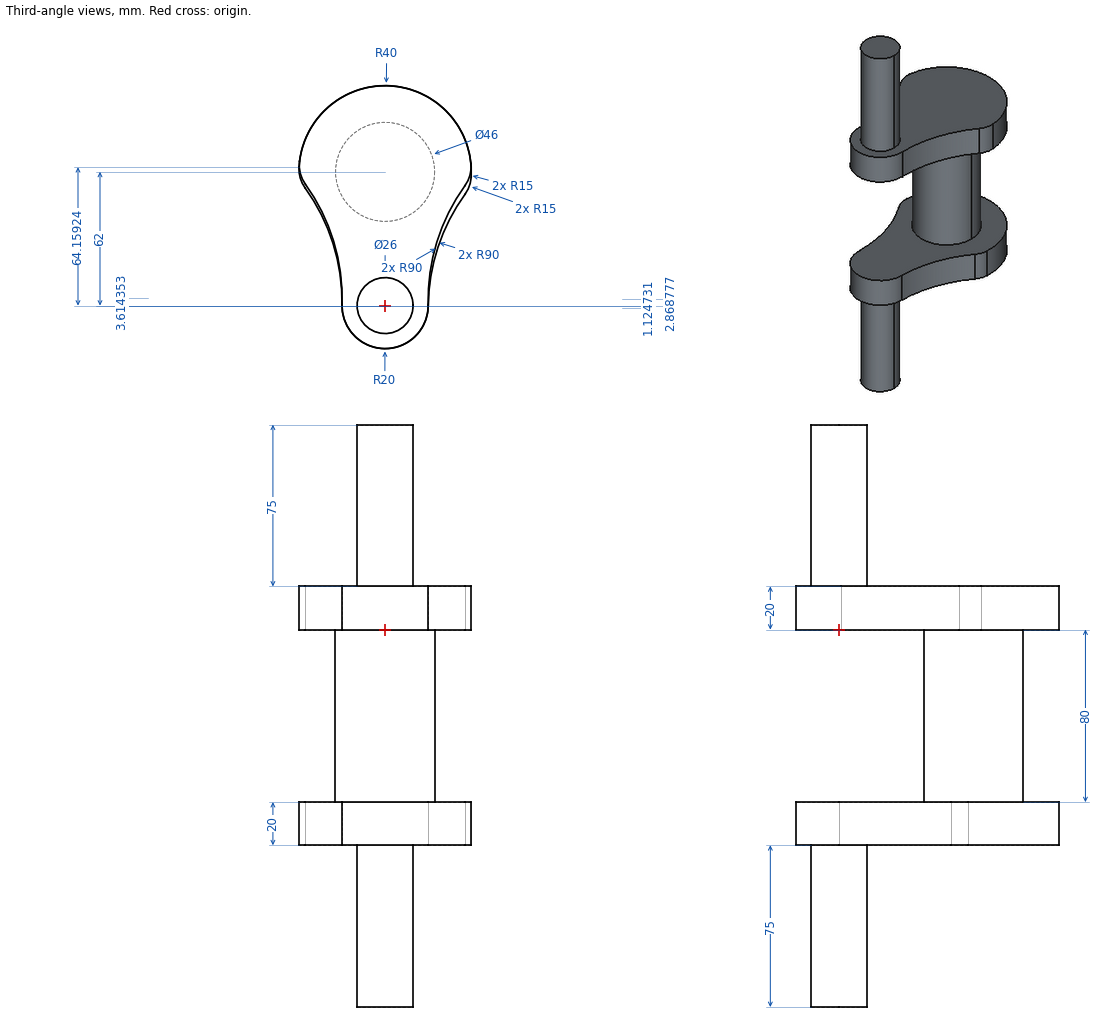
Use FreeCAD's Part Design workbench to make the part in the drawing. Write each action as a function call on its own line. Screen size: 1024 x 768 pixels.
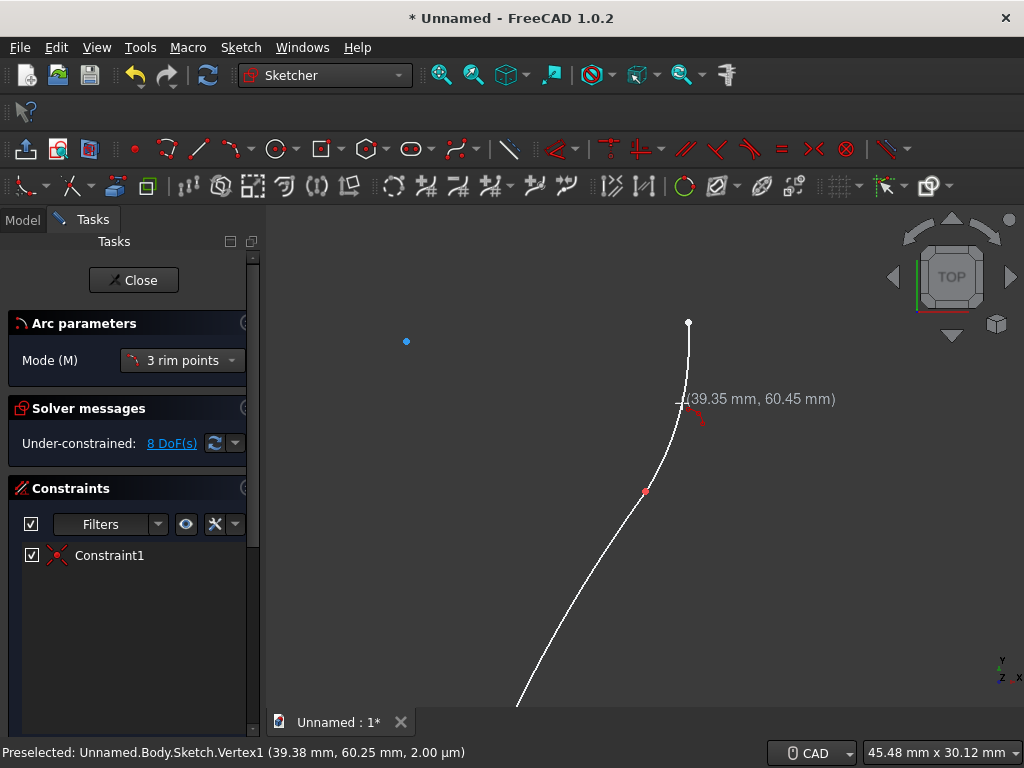
scroll(685, 402, down, 9)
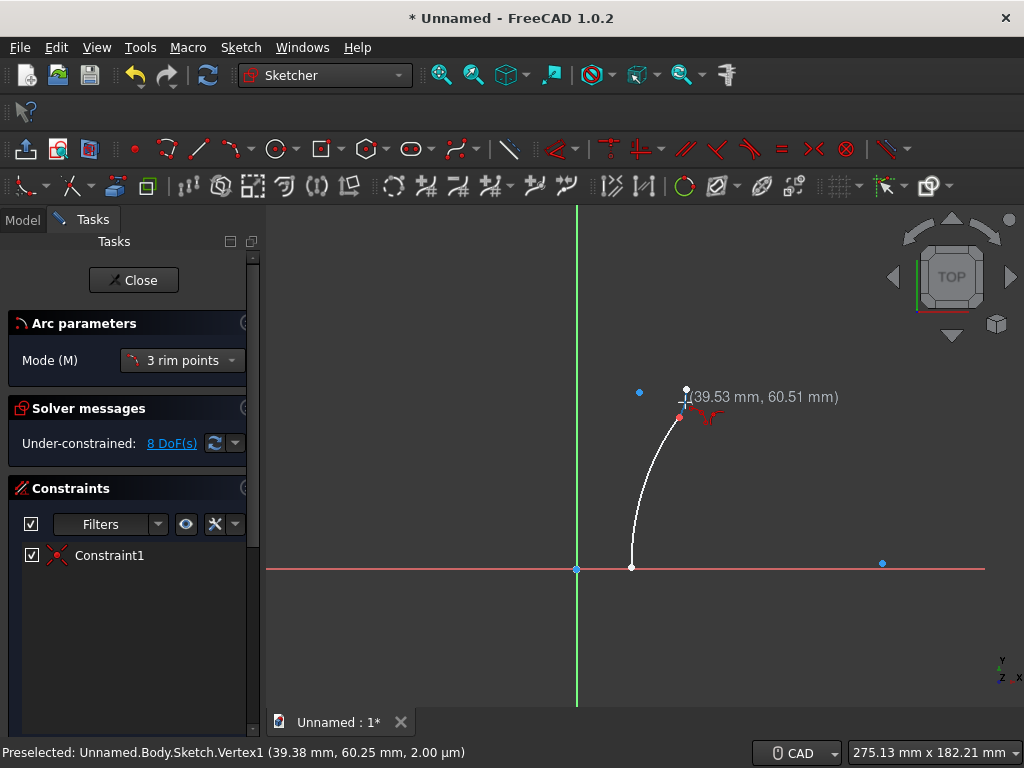
click(686, 389)
click(467, 385)
click(610, 293)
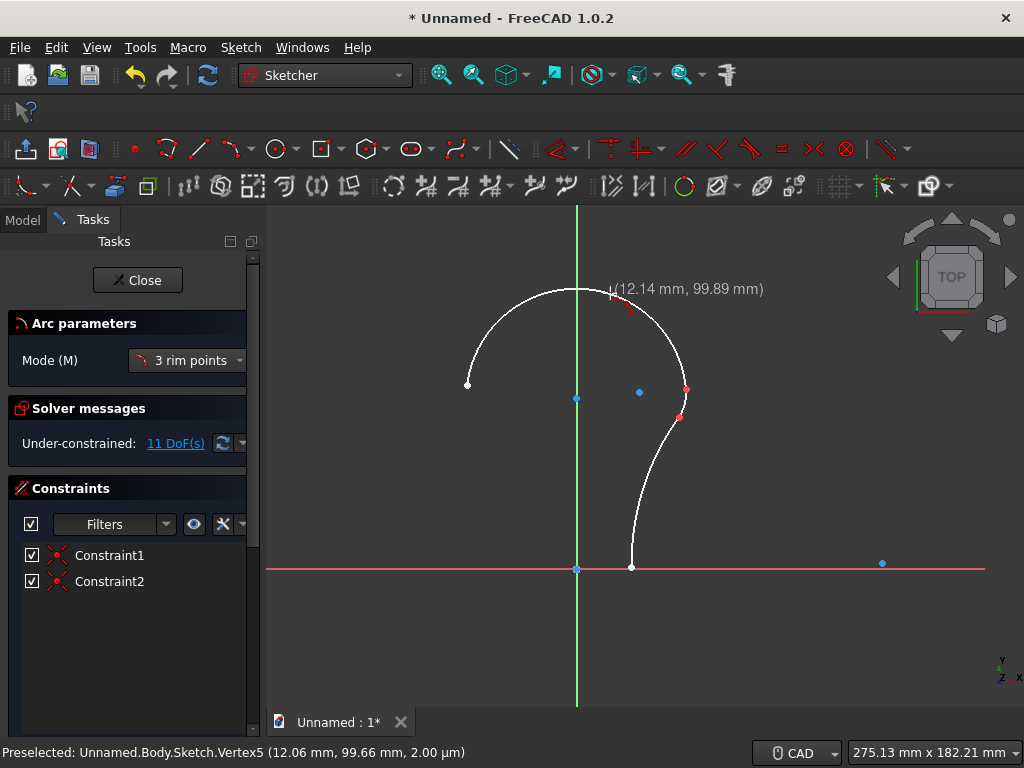
click(467, 386)
click(475, 414)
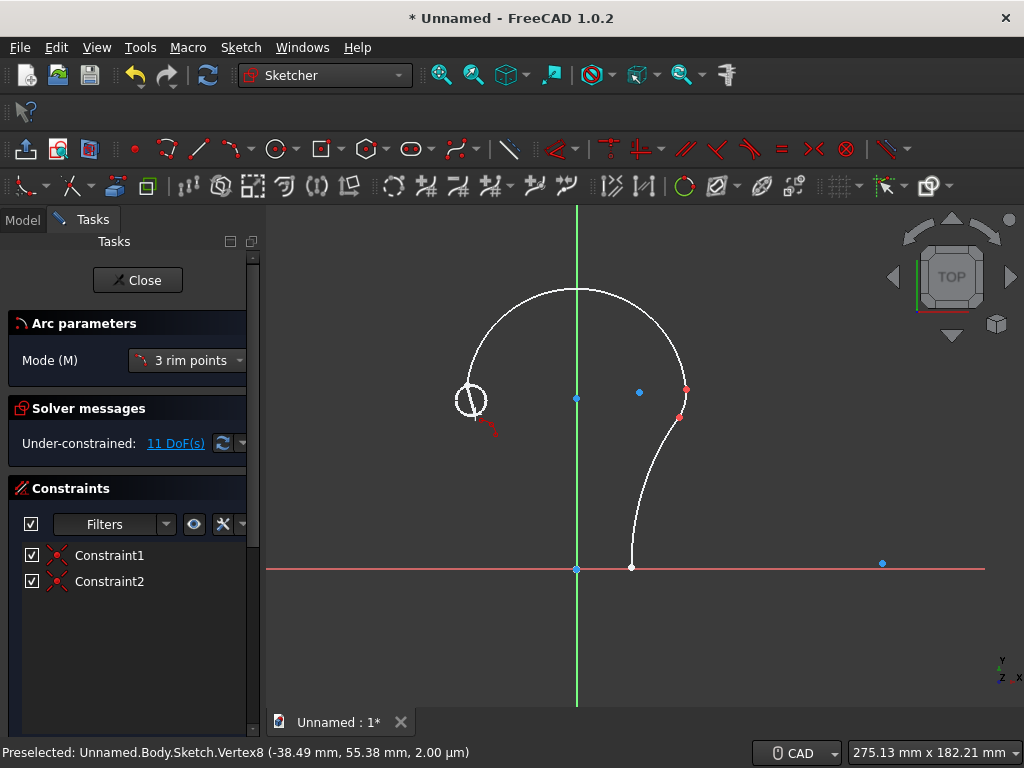
scroll(468, 400, up, 9)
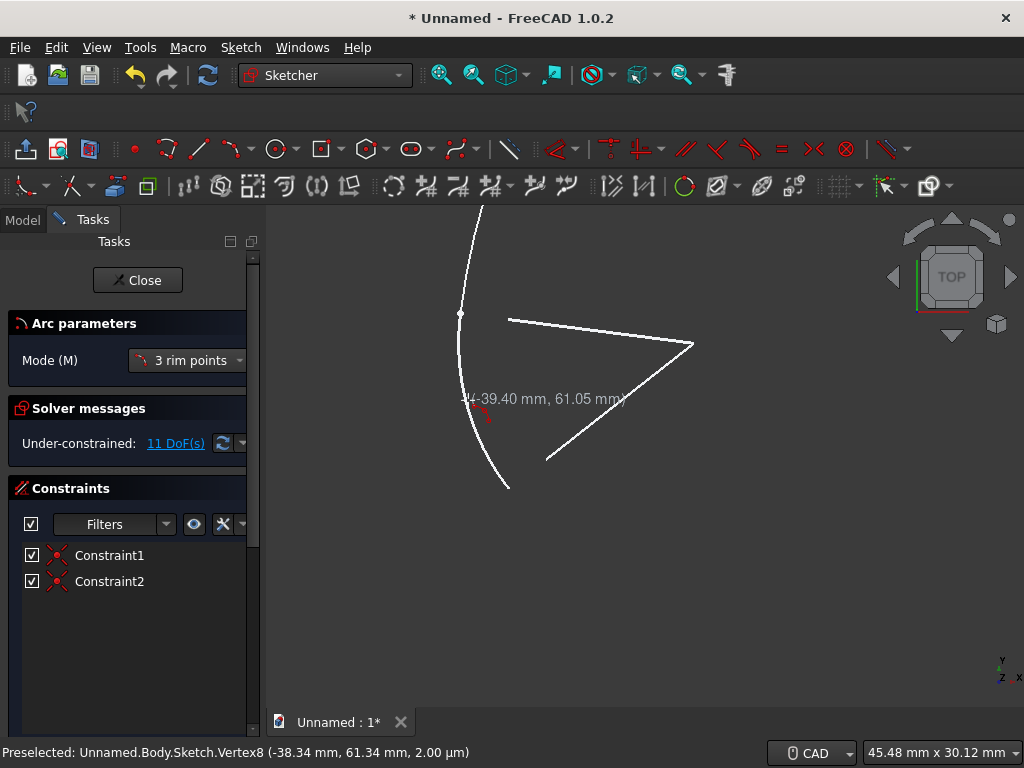
click(468, 399)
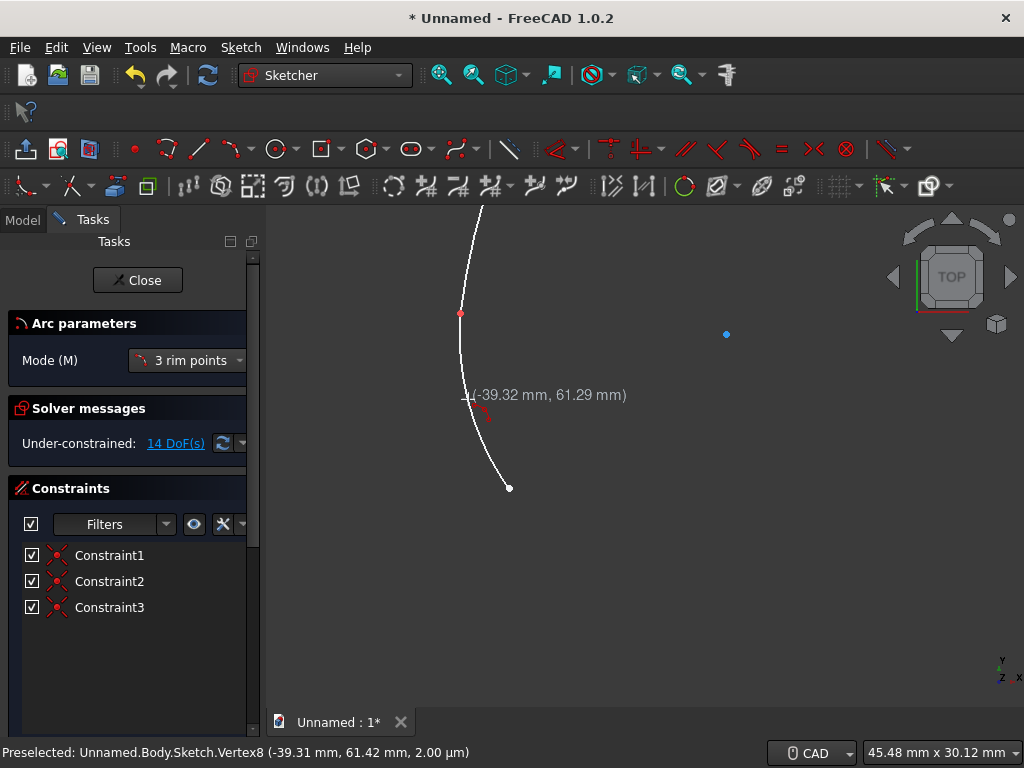
scroll(468, 400, down, 9)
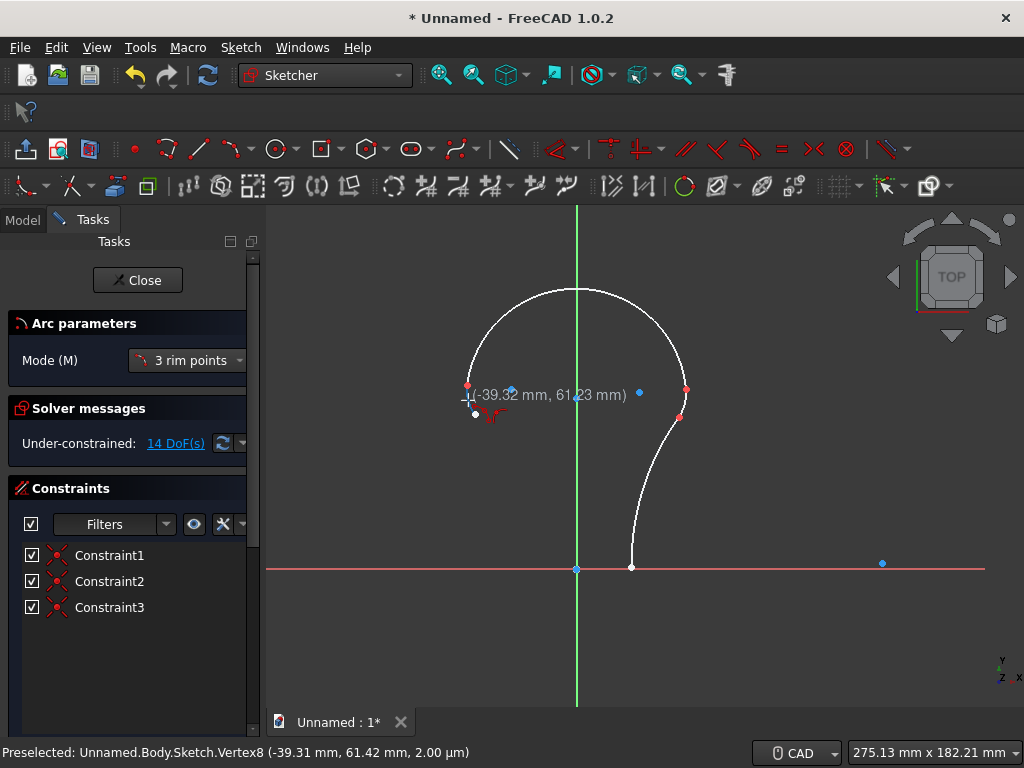
click(475, 415)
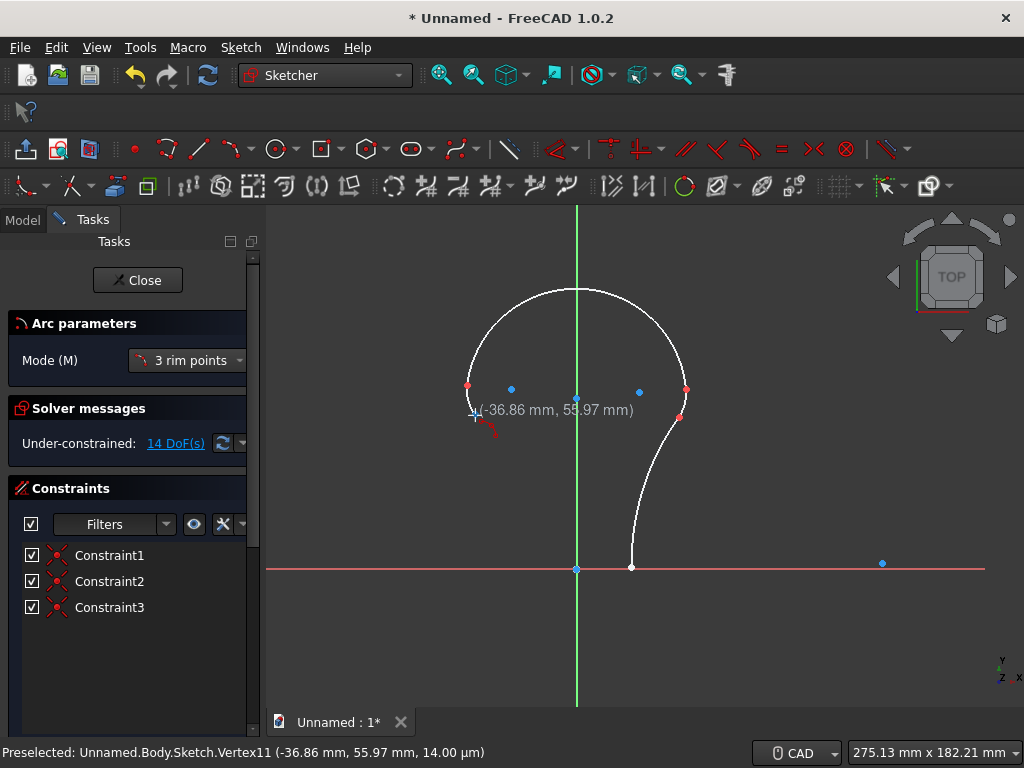
scroll(521, 567, up, 11)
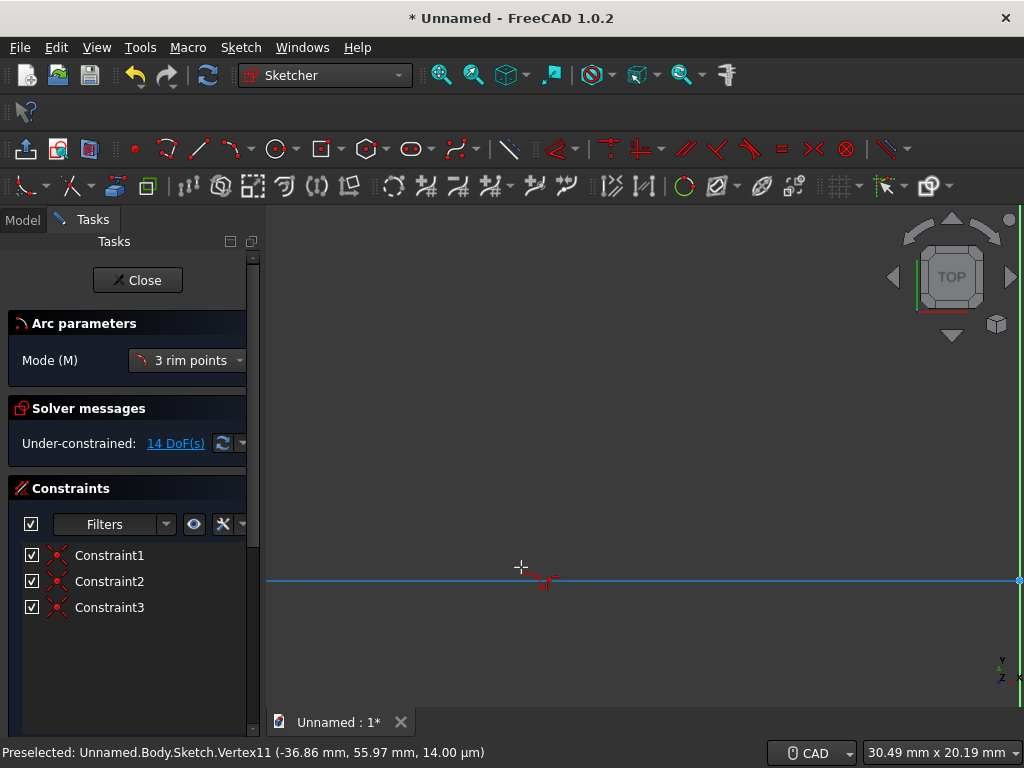
click(523, 565)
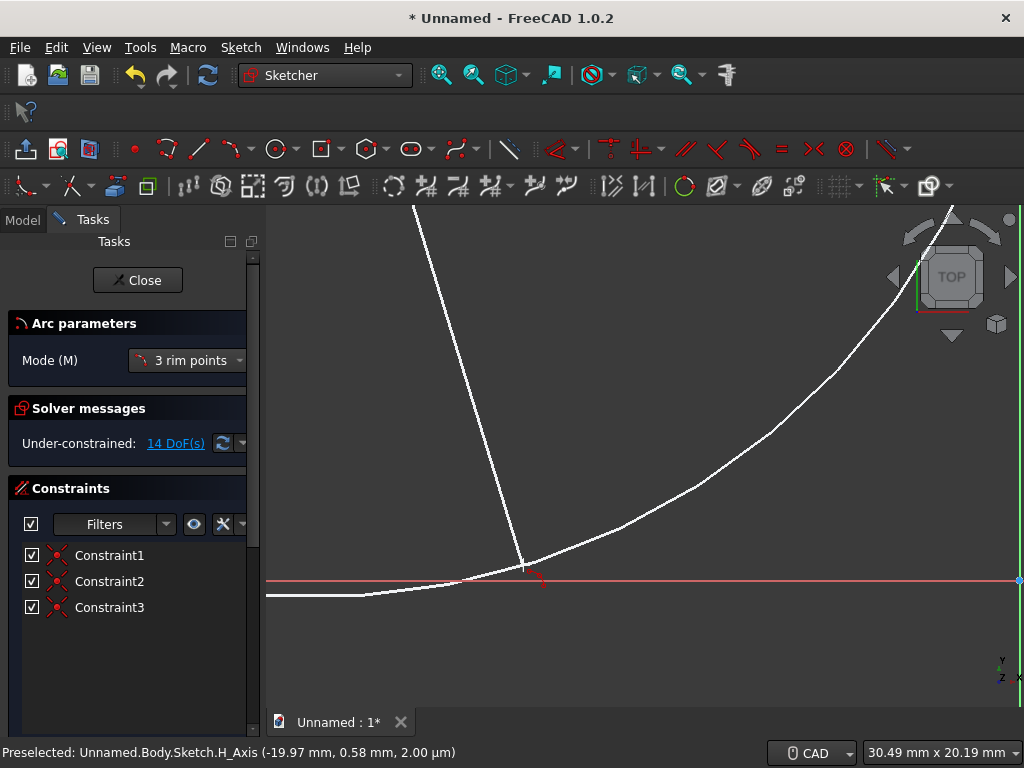
scroll(521, 567, down, 11)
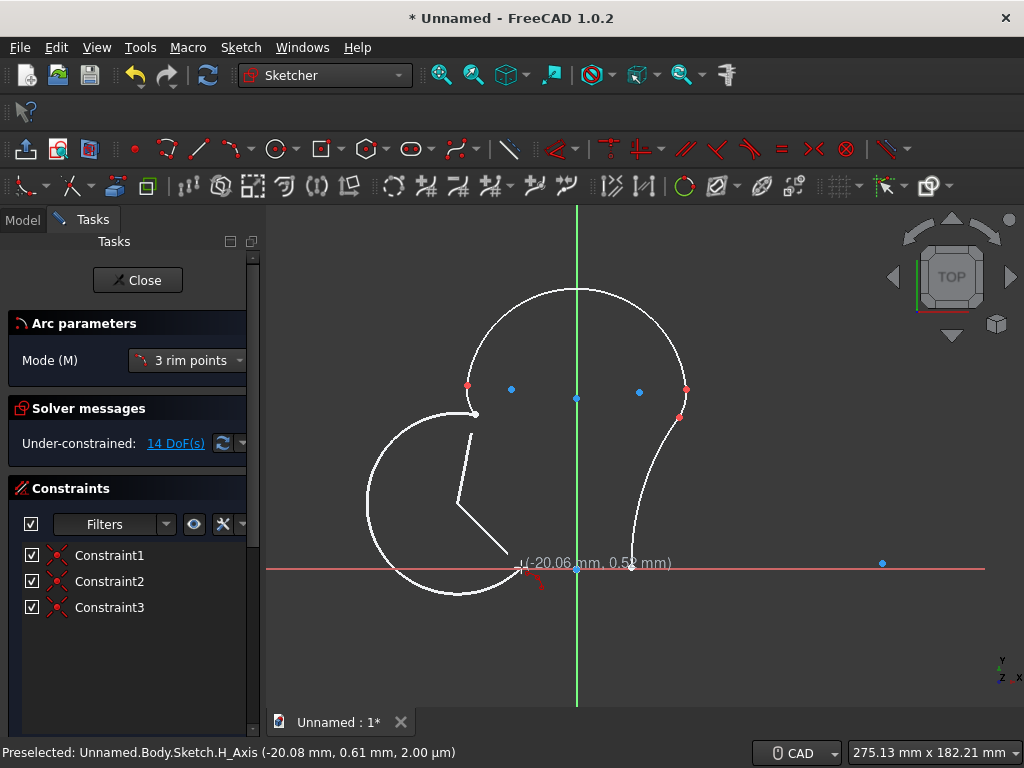
click(511, 487)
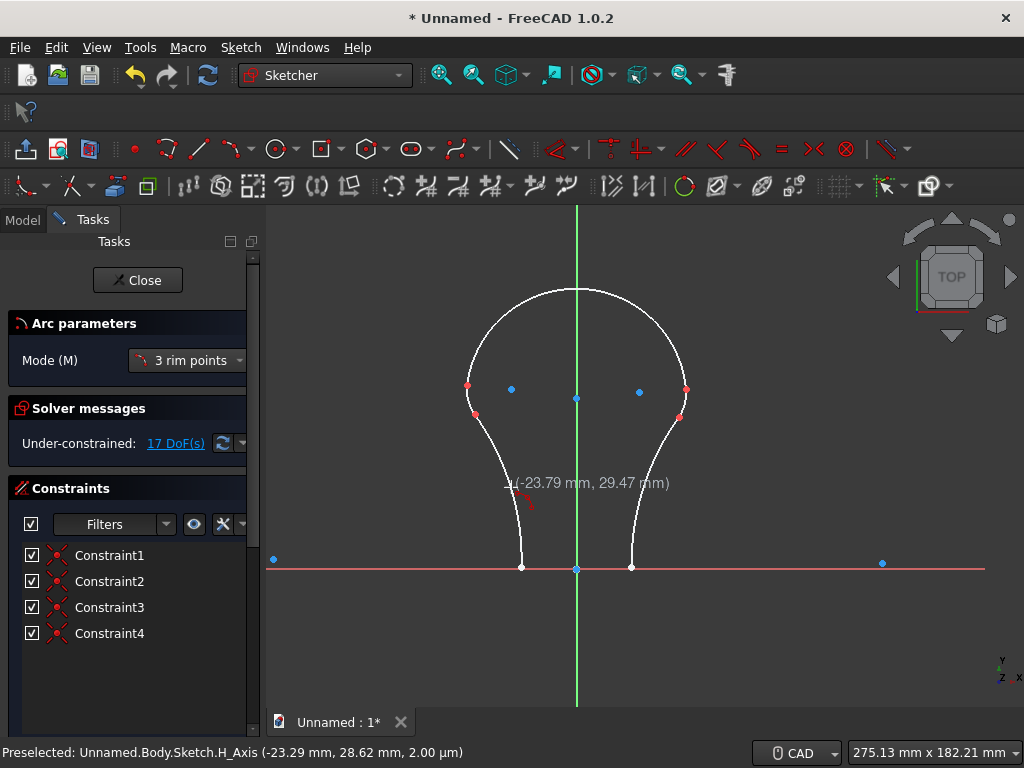
scroll(521, 567, up, 11)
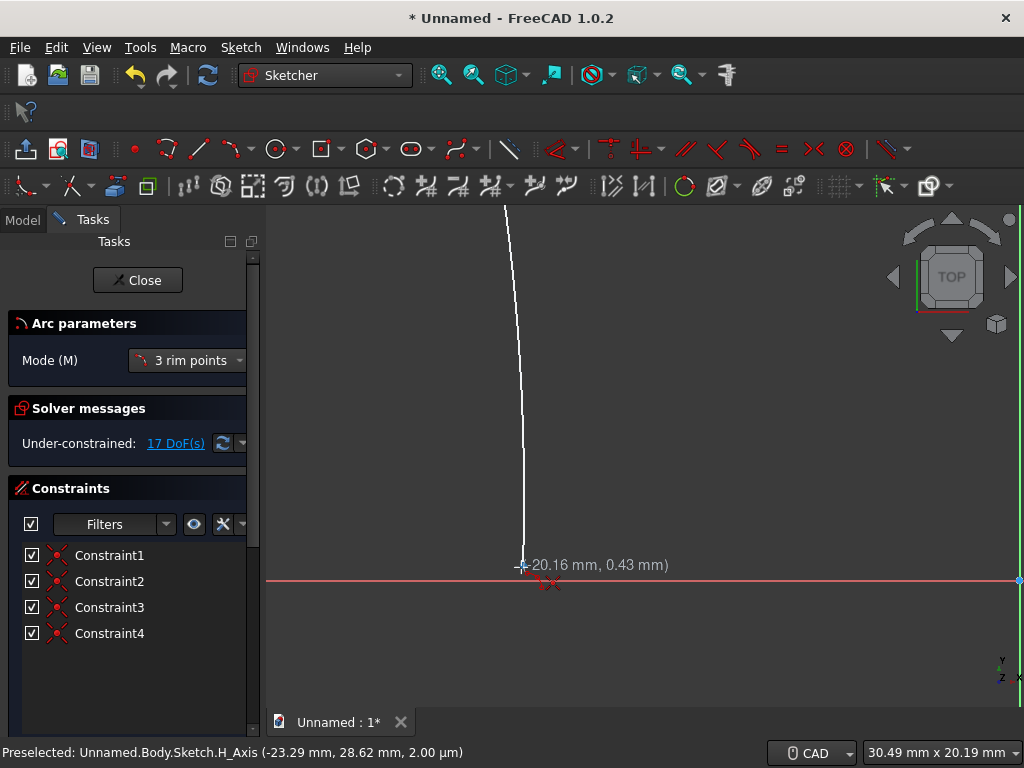
click(523, 566)